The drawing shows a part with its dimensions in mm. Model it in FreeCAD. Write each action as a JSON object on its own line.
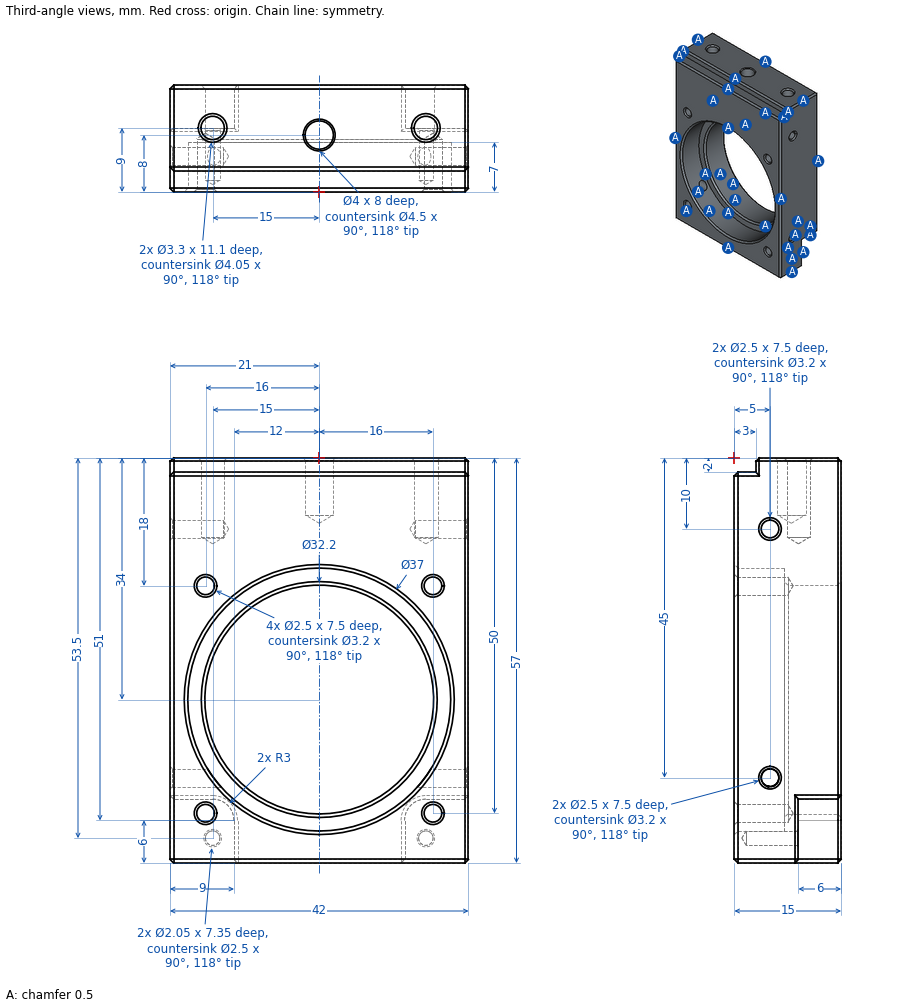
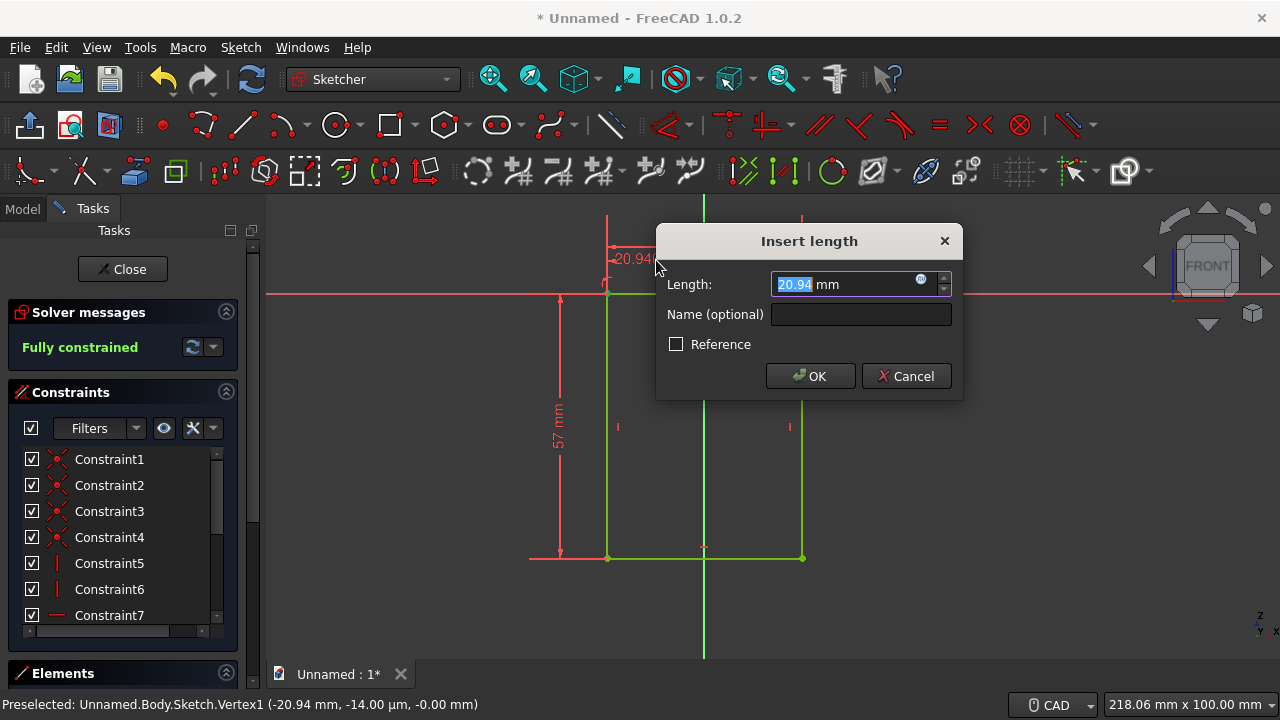
{"action": "type", "text": "21"}
{"action": "key", "text": "Return"}
{"action": "key", "text": "Escape"}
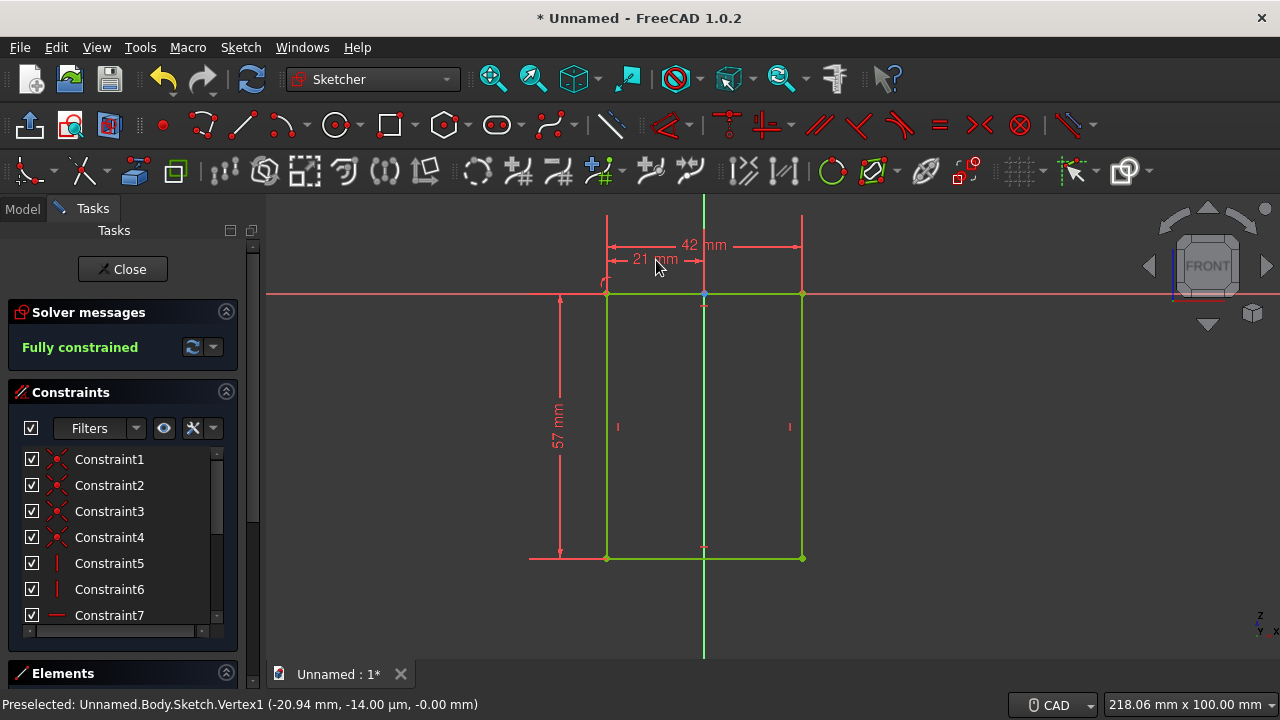
{"action": "left_click", "coordinate": [123, 269]}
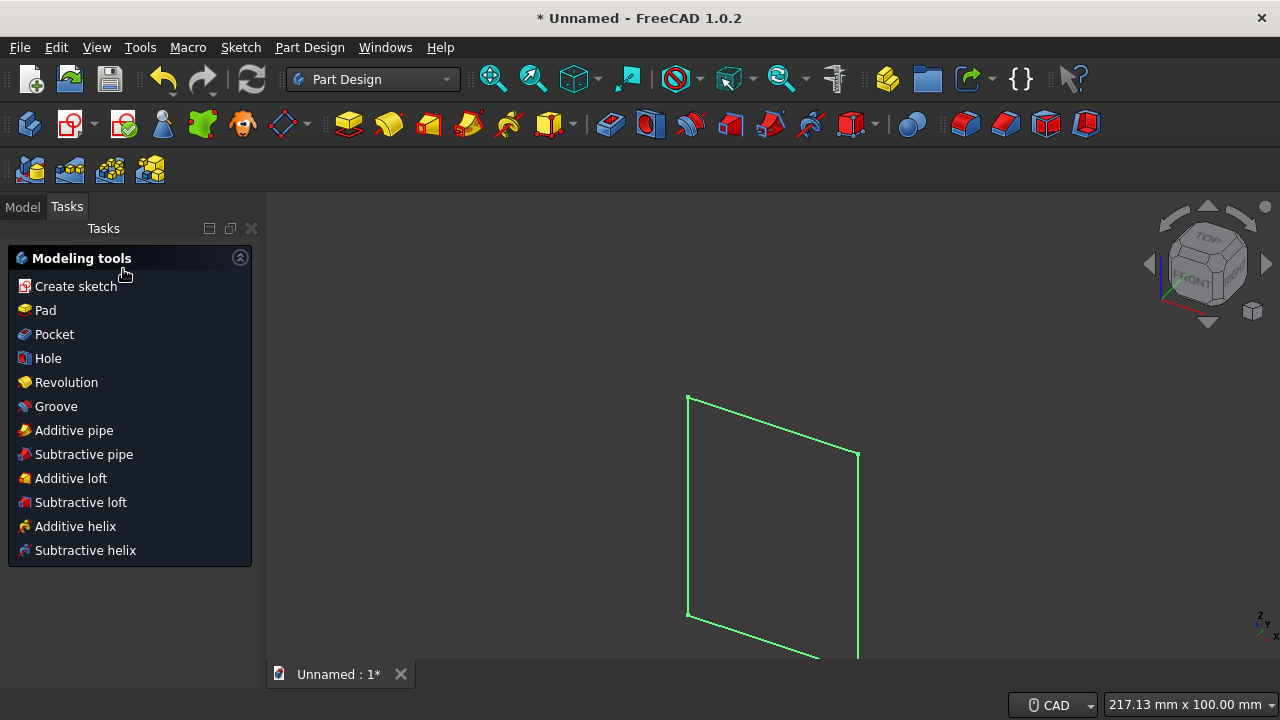
{"action": "left_click", "coordinate": [350, 124]}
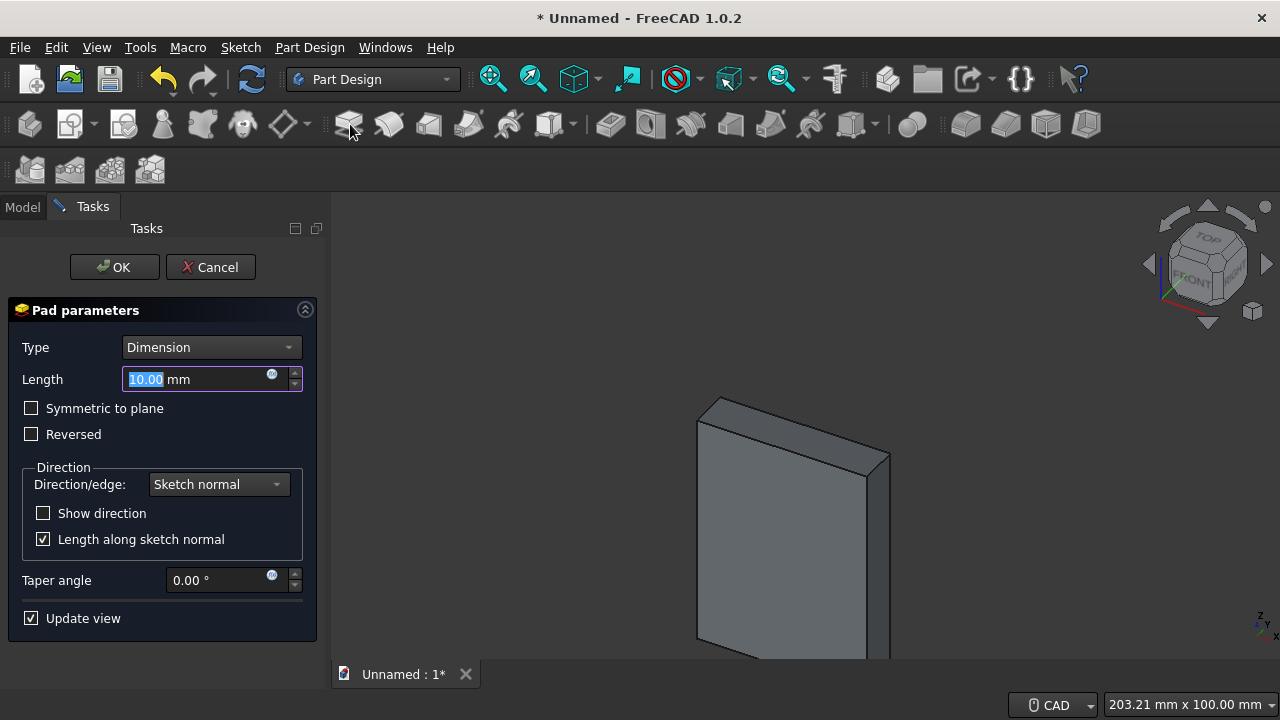
{"action": "type", "text": "15"}
{"action": "key", "text": "Tab"}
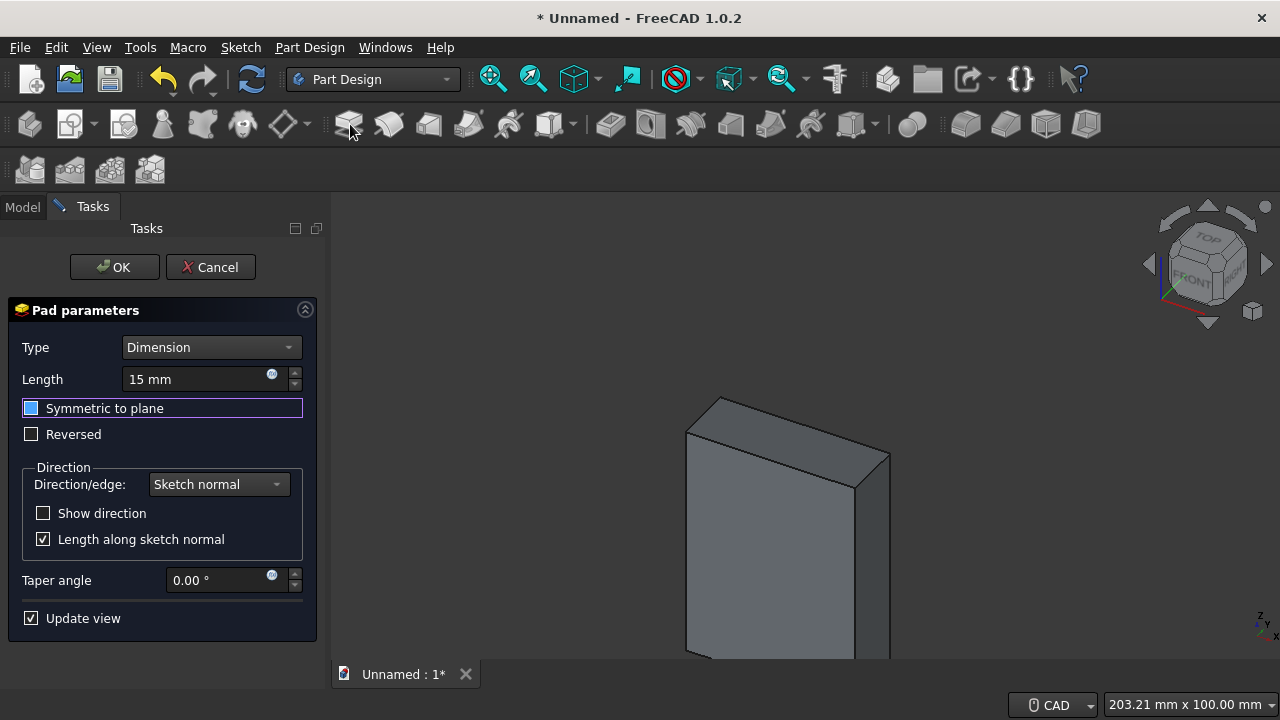
{"action": "left_click", "coordinate": [30, 434]}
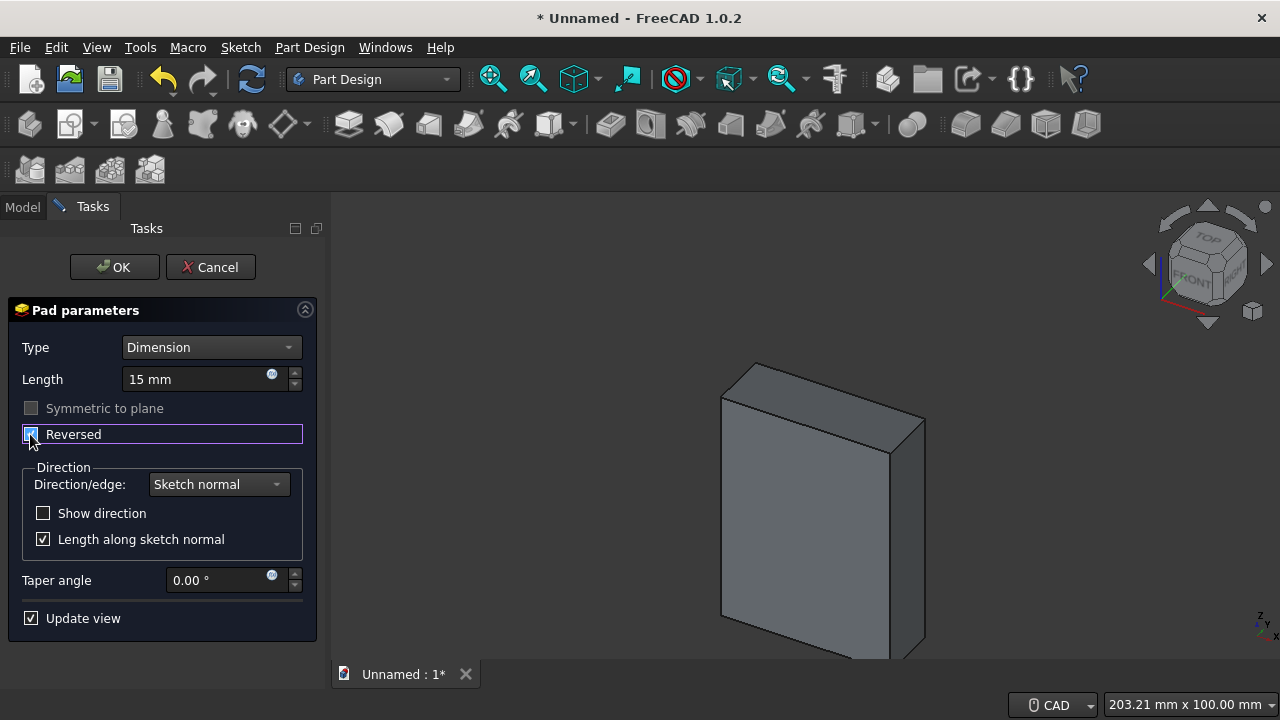
{"action": "left_click", "coordinate": [115, 267]}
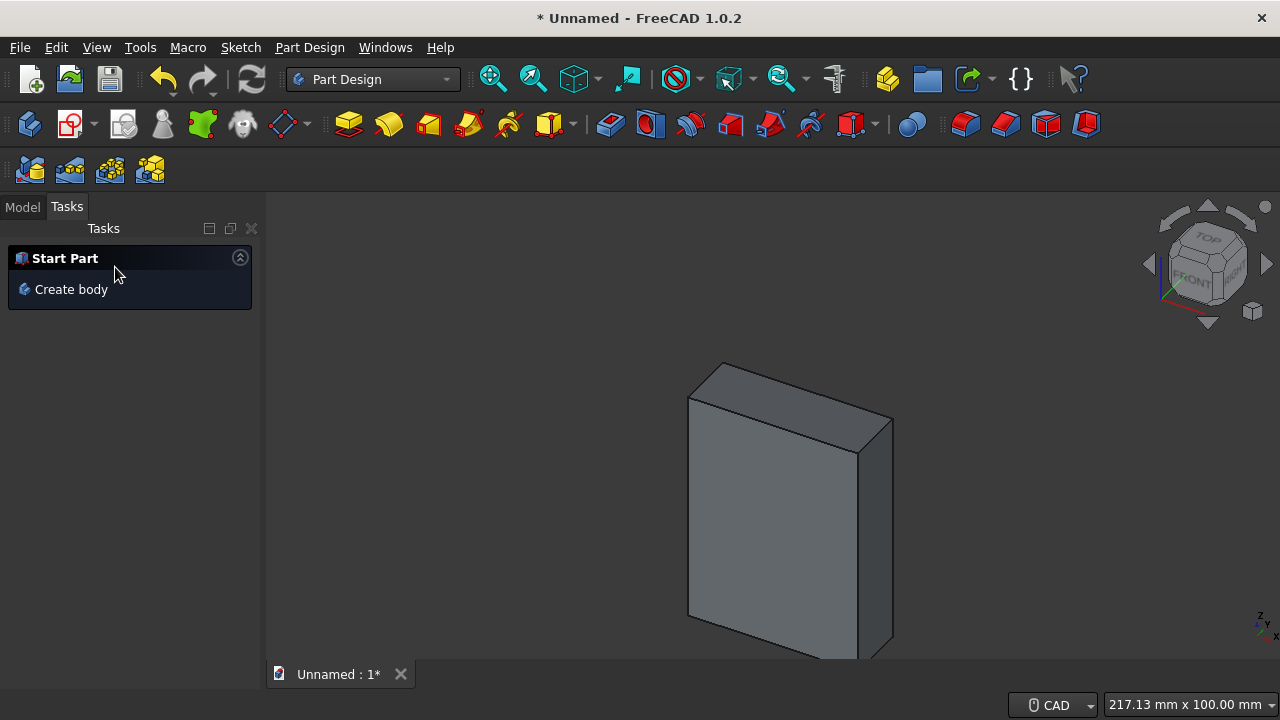
{"action": "left_click", "coordinate": [494, 80]}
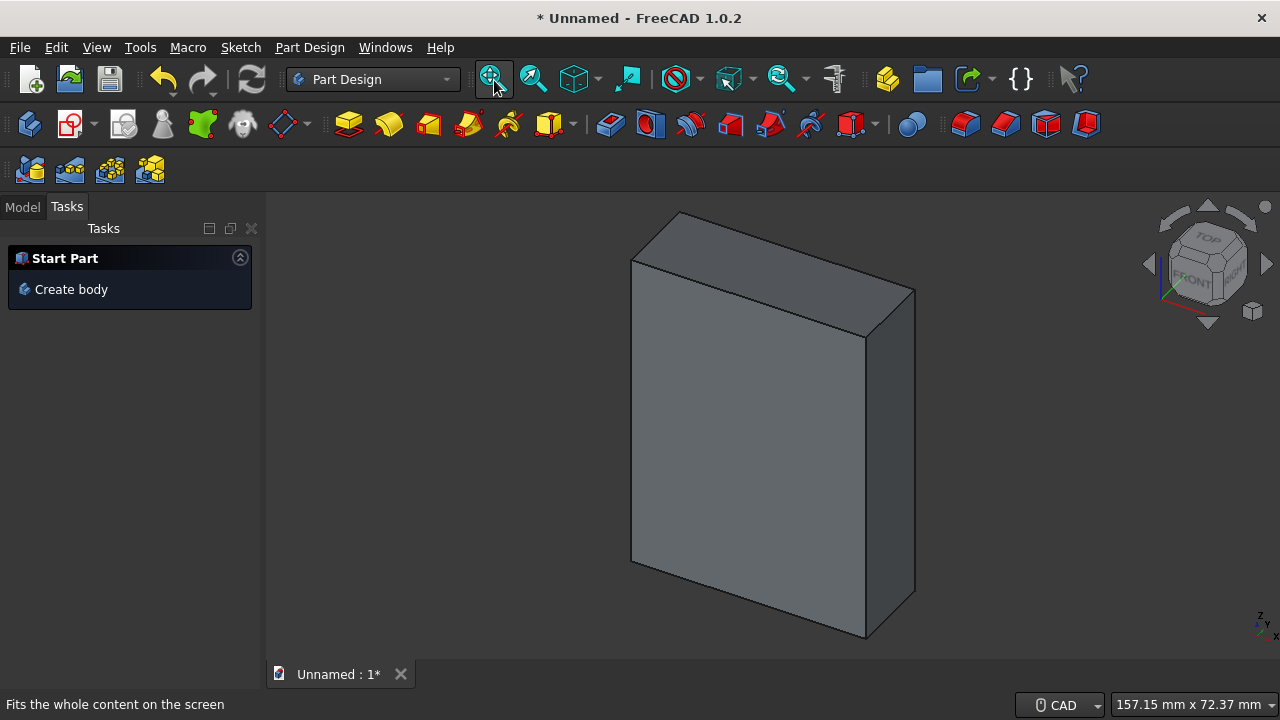
{"action": "left_click", "coordinate": [749, 449]}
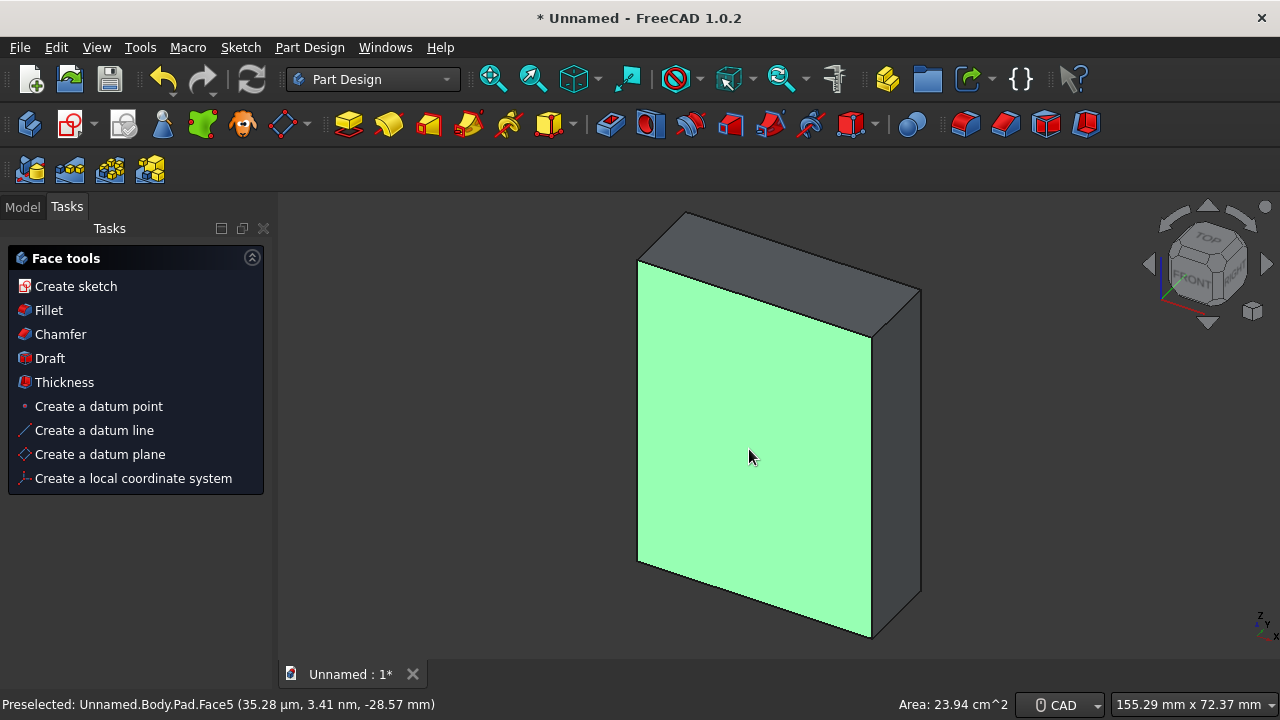
{"action": "left_click", "coordinate": [70, 124]}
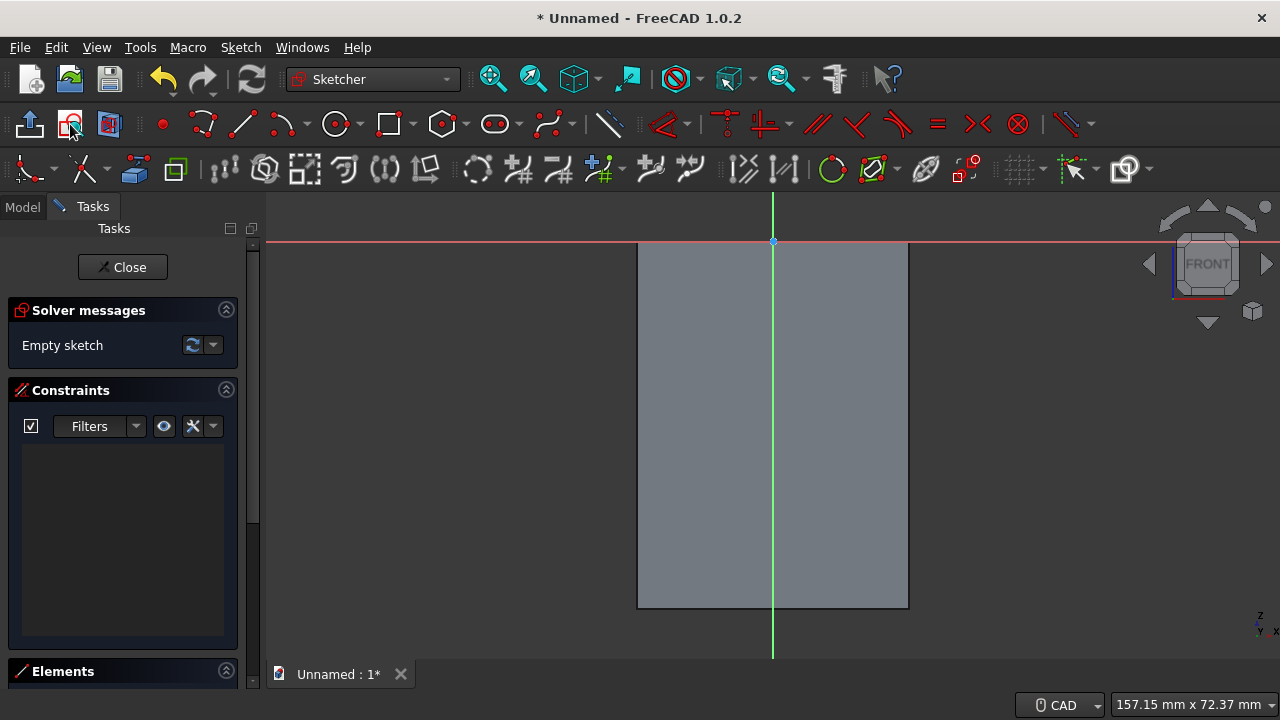
{"action": "scroll", "coordinate": [395, 491], "scroll_direction": "down", "scroll_amount": 1}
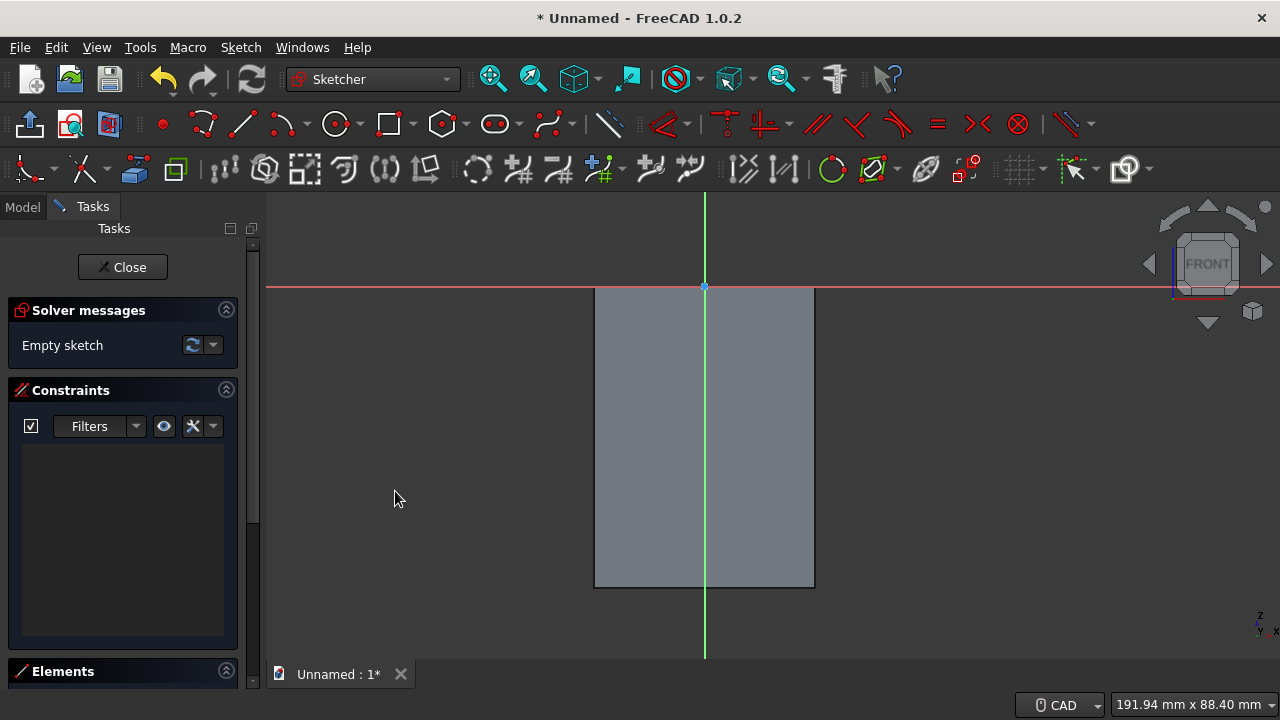
{"action": "key", "text": "g c"}